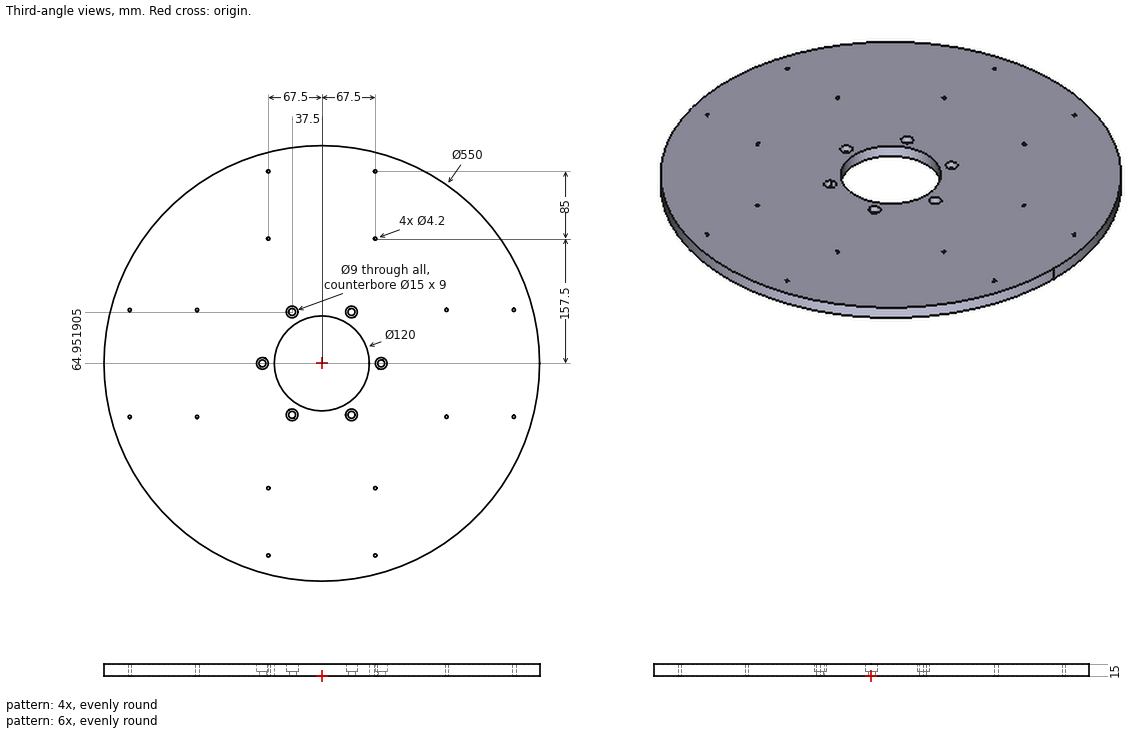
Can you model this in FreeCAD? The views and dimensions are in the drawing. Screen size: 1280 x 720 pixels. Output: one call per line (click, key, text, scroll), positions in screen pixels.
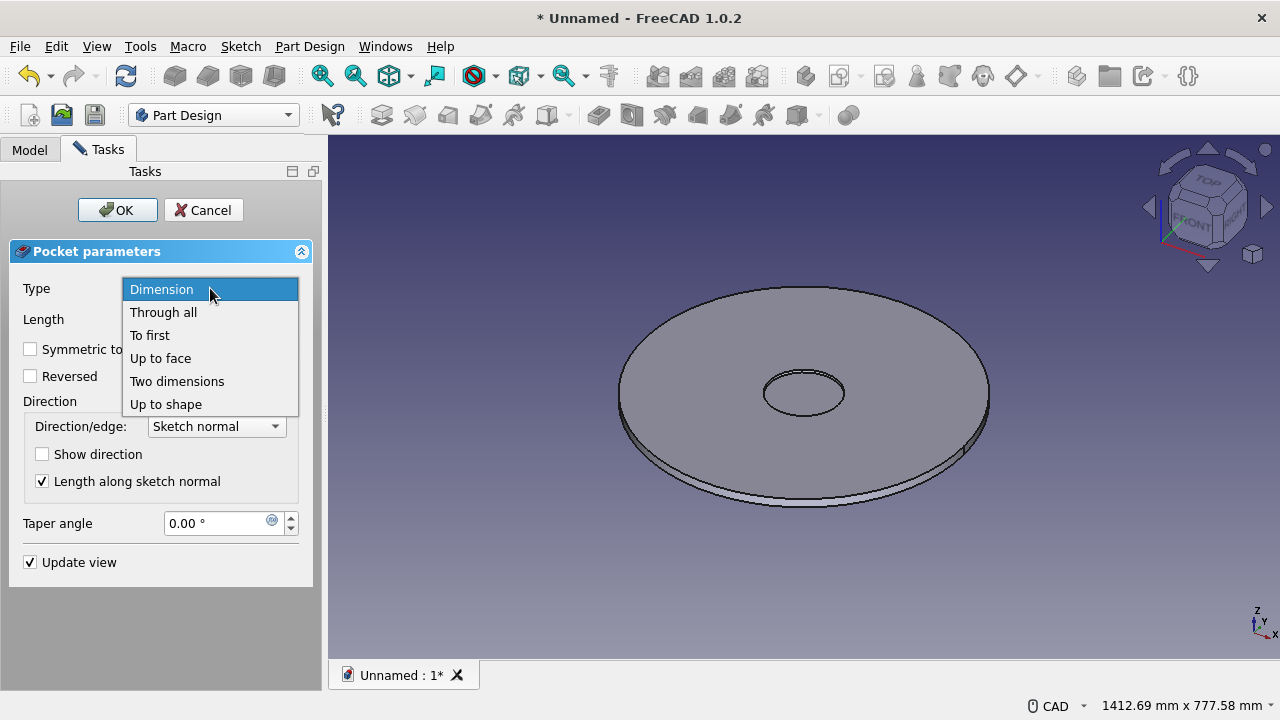
click(208, 312)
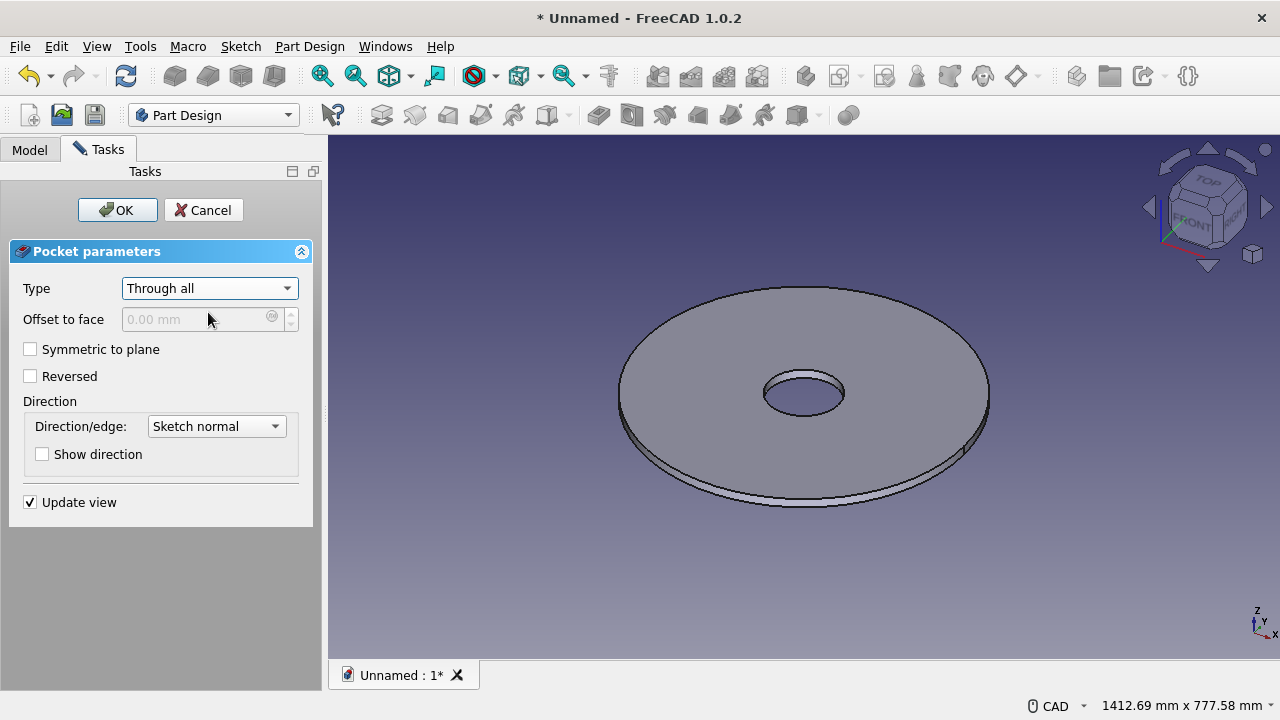
click(118, 210)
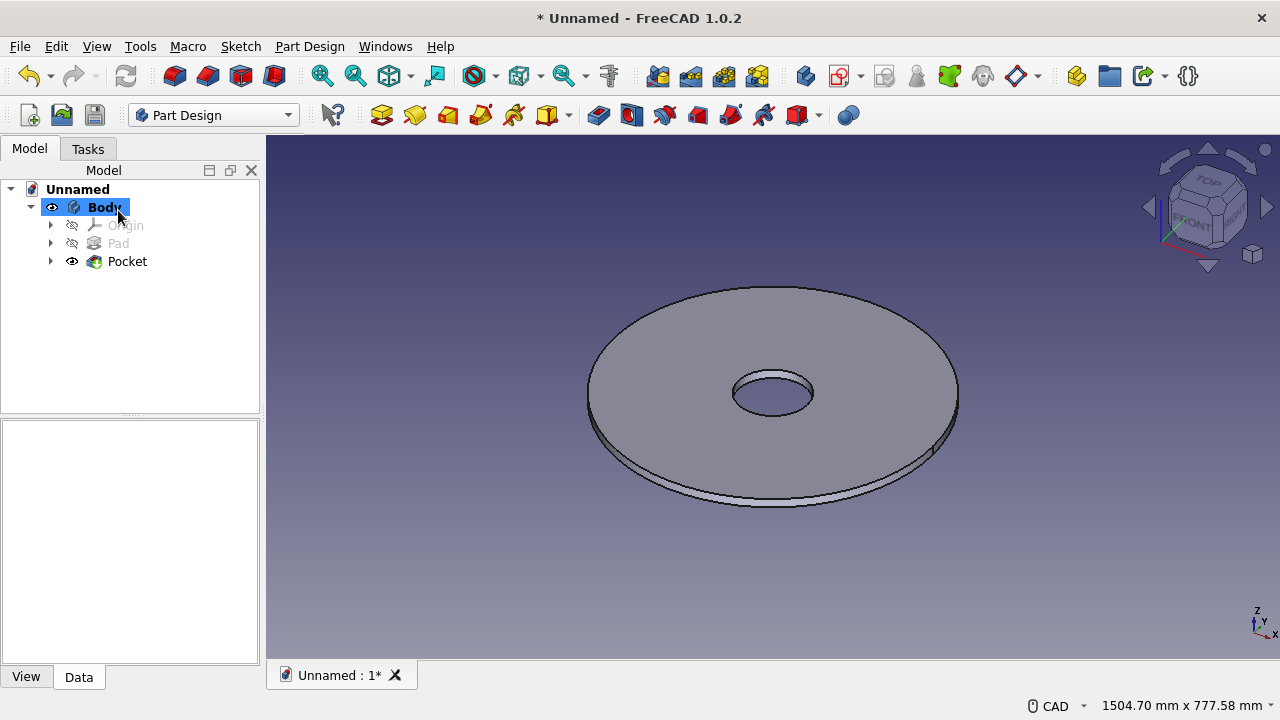
click(766, 460)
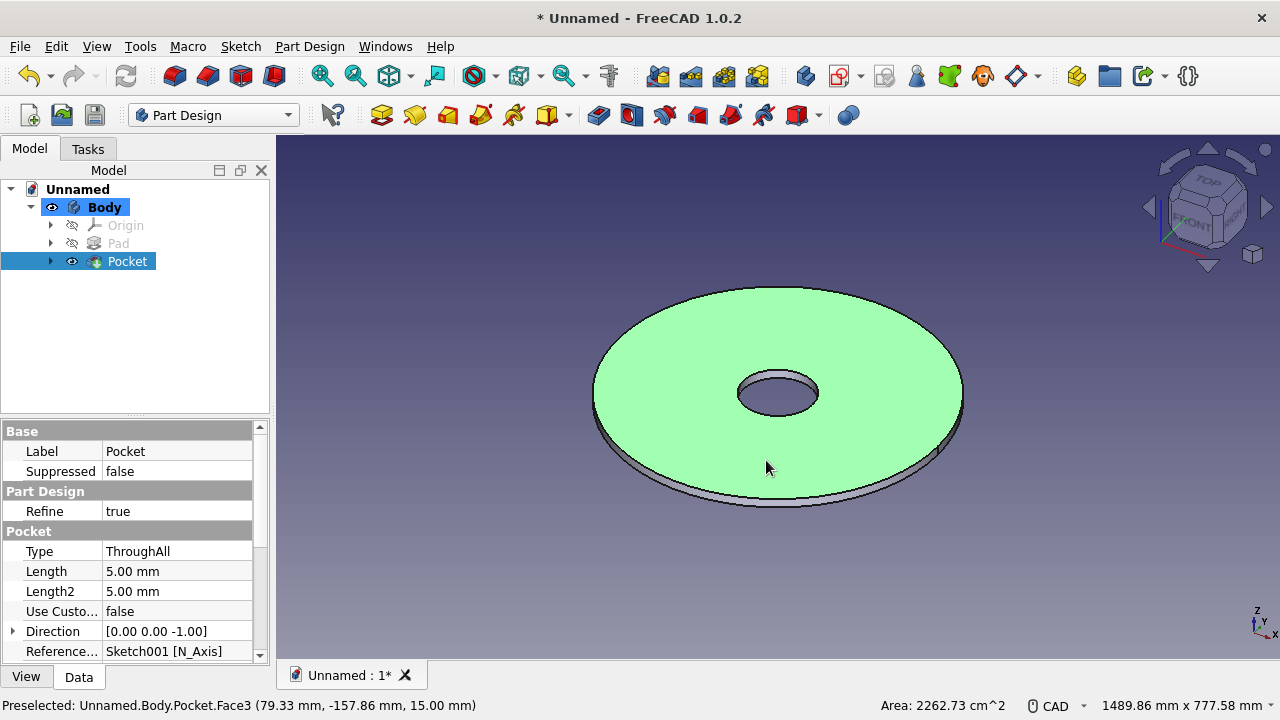
click(838, 76)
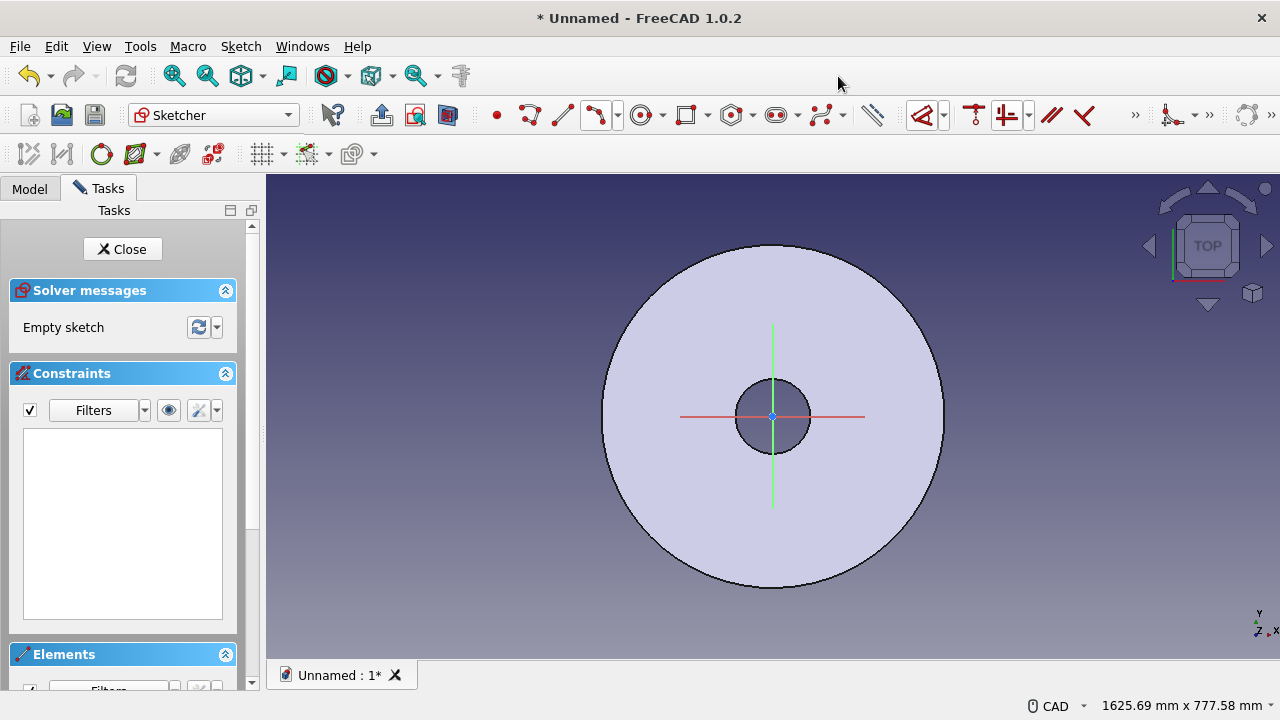
scroll(856, 247, up, 3)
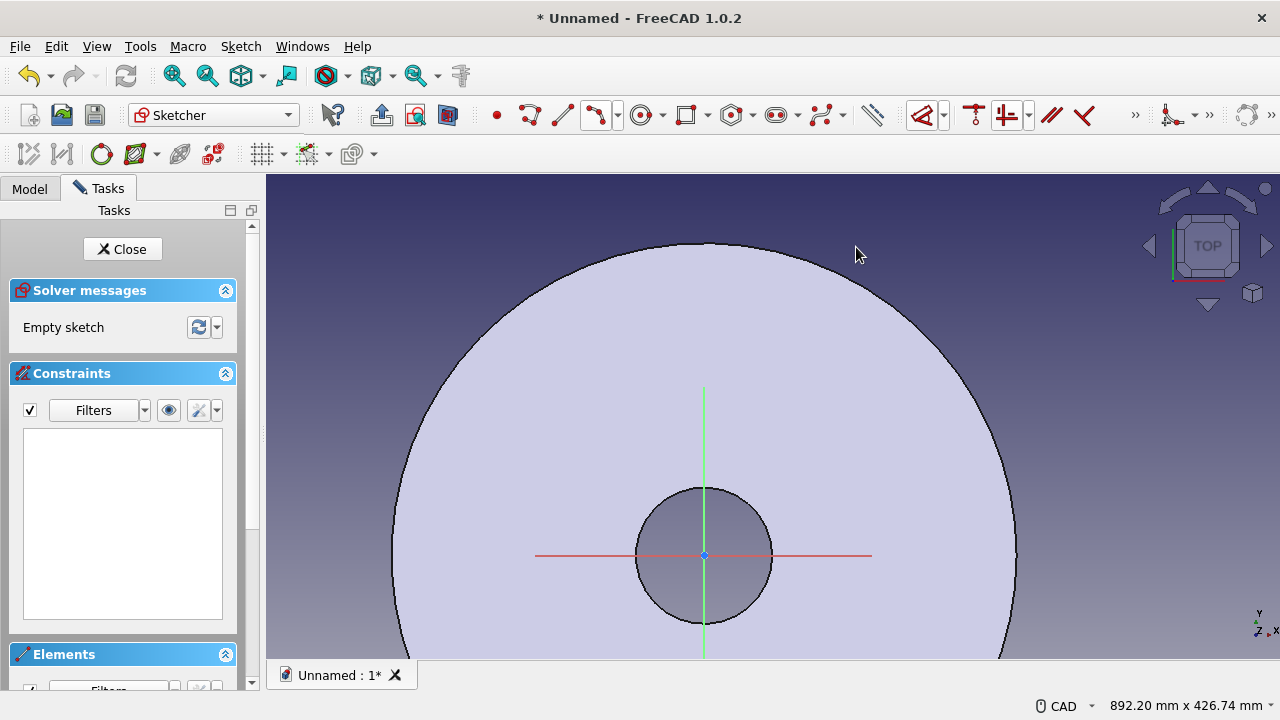
click(640, 116)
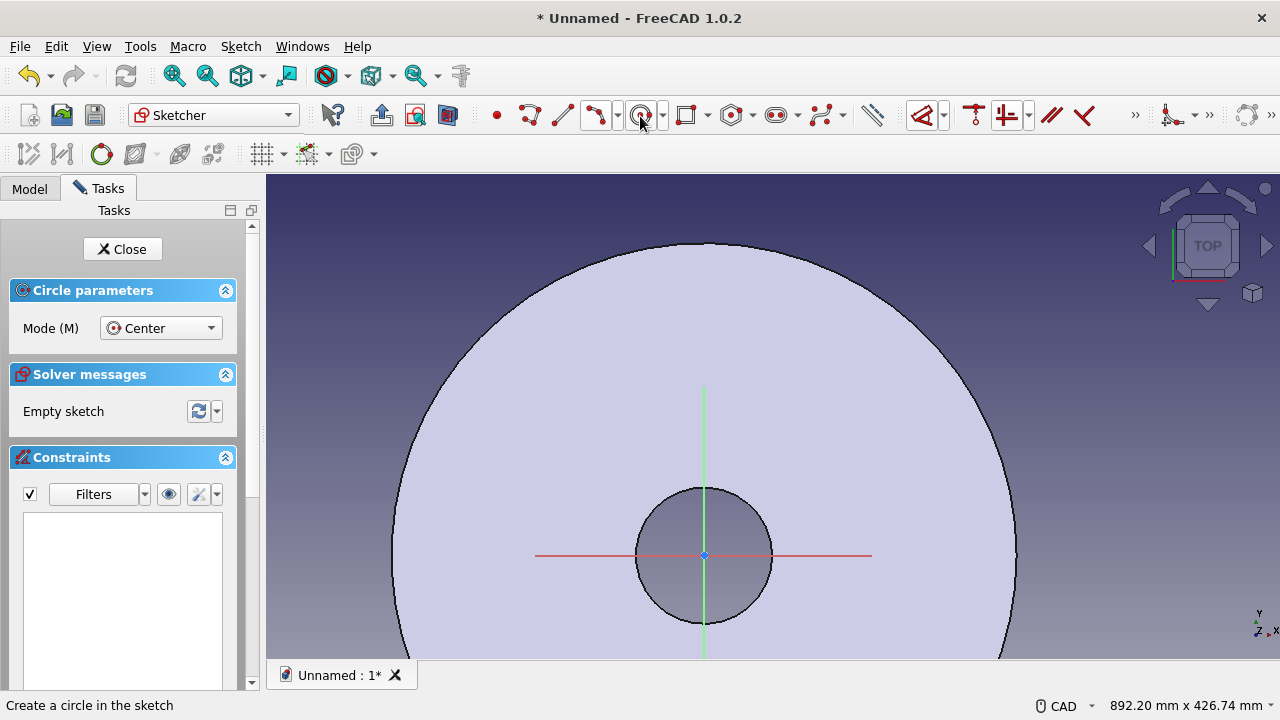
scroll(781, 377, up, 12)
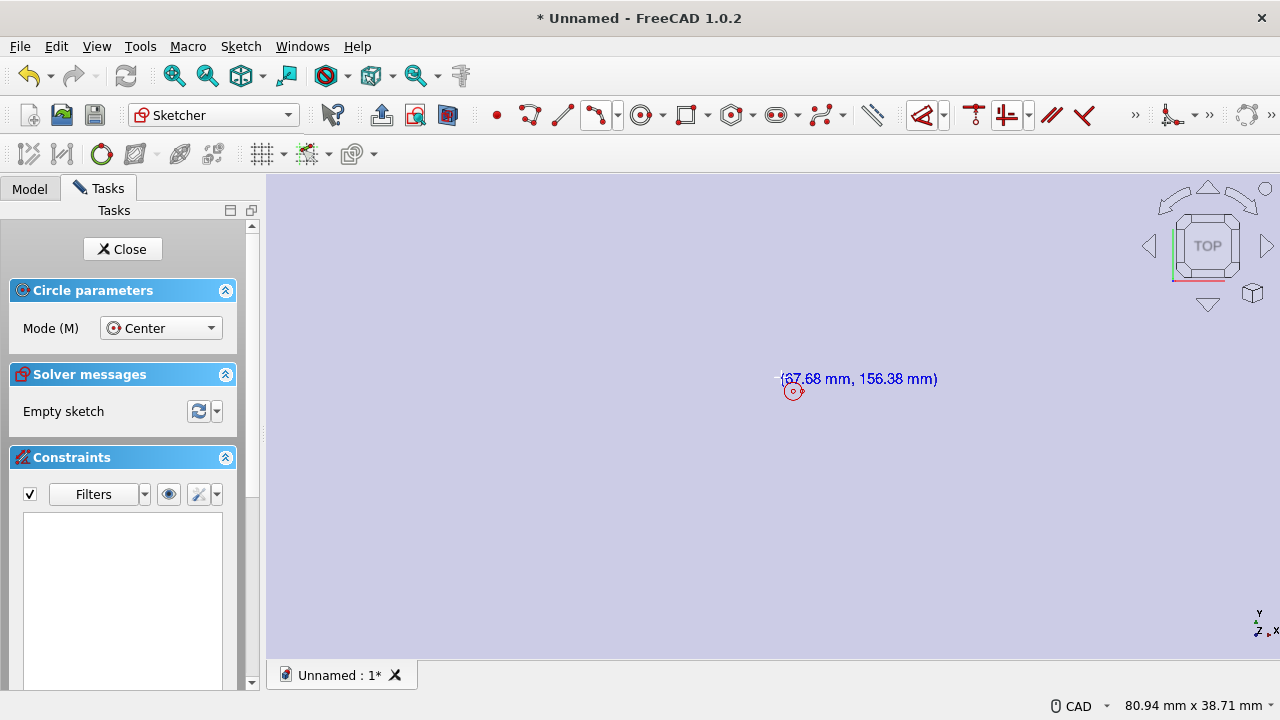
scroll(782, 377, down, 12)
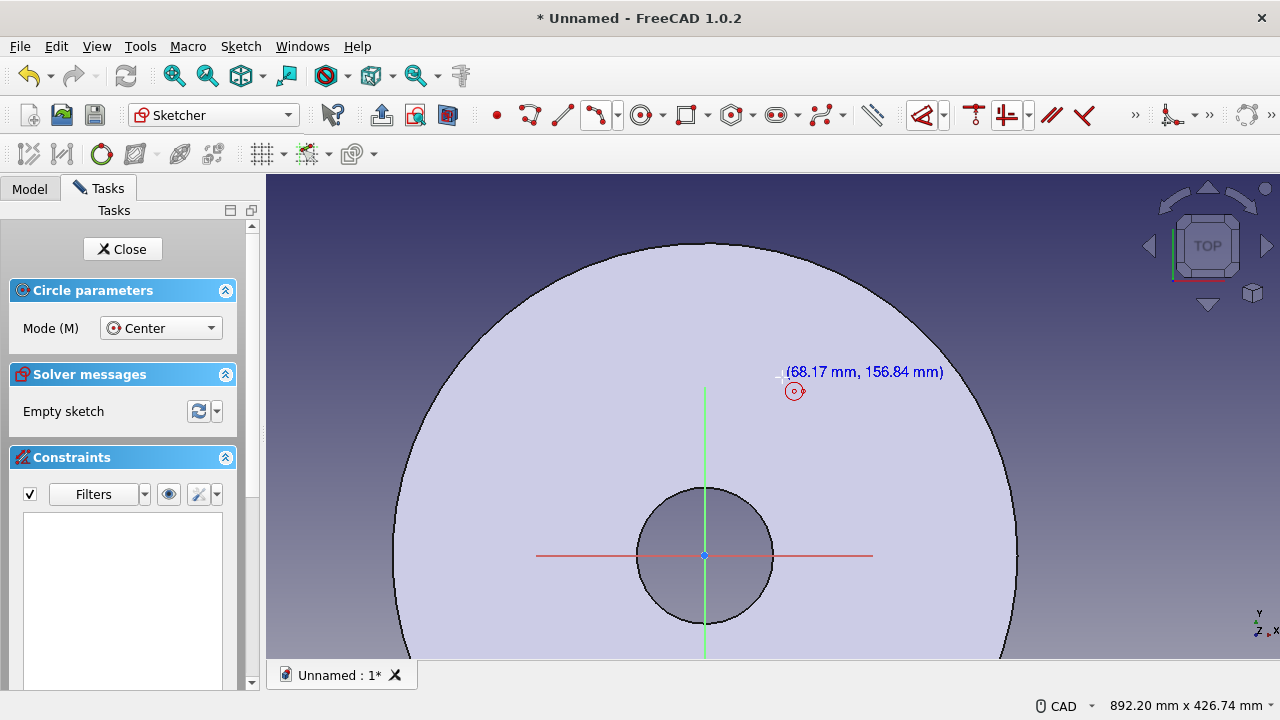
click(782, 377)
move(783, 375)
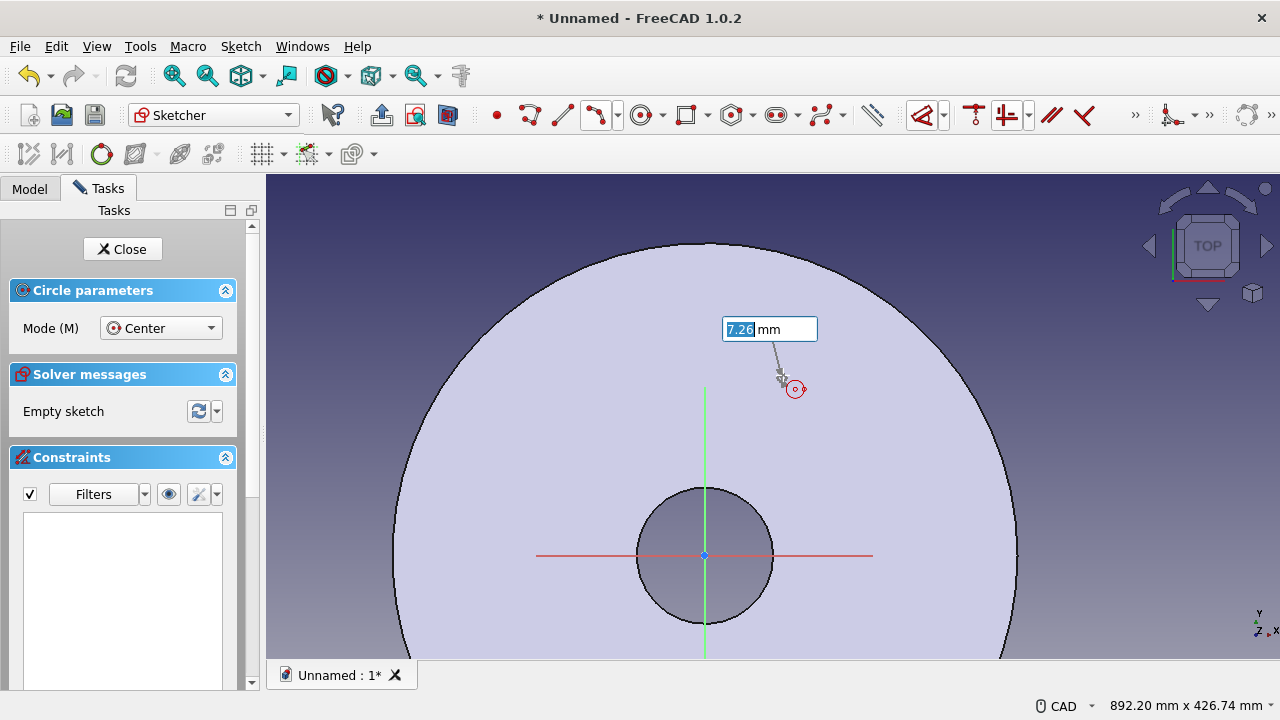
text(4.2)
key(Return)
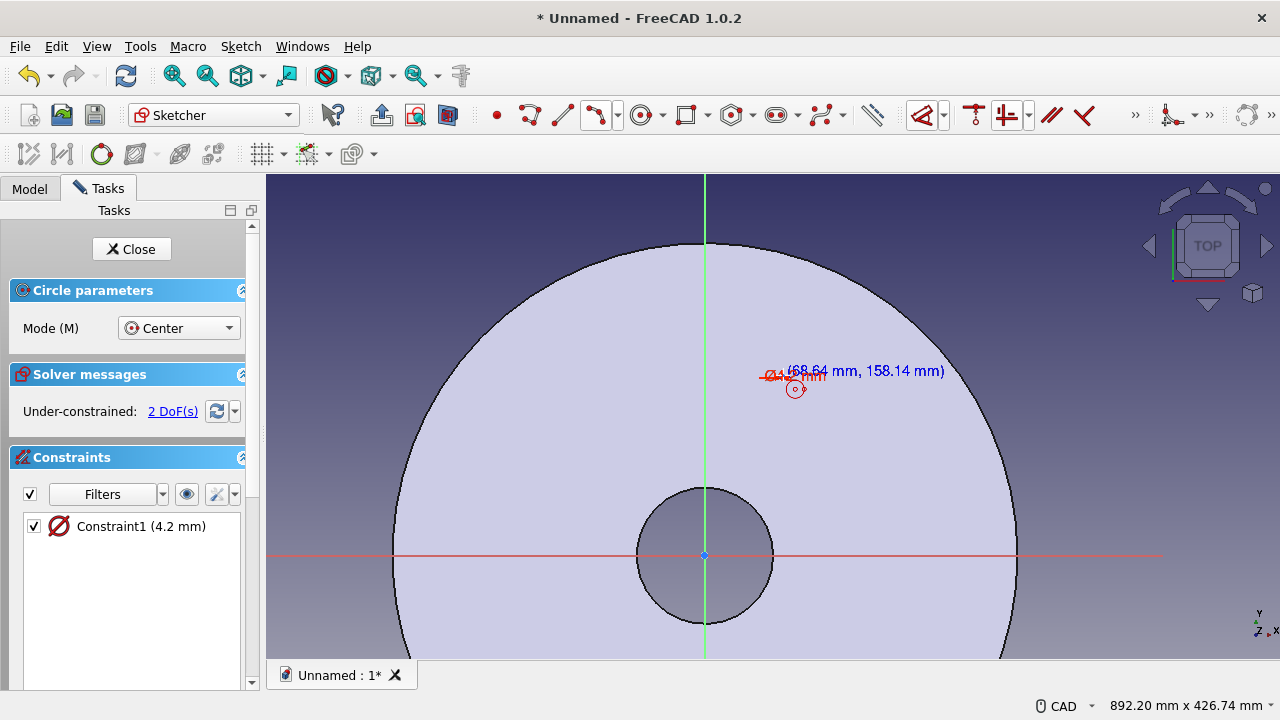
scroll(782, 280, up, 12)